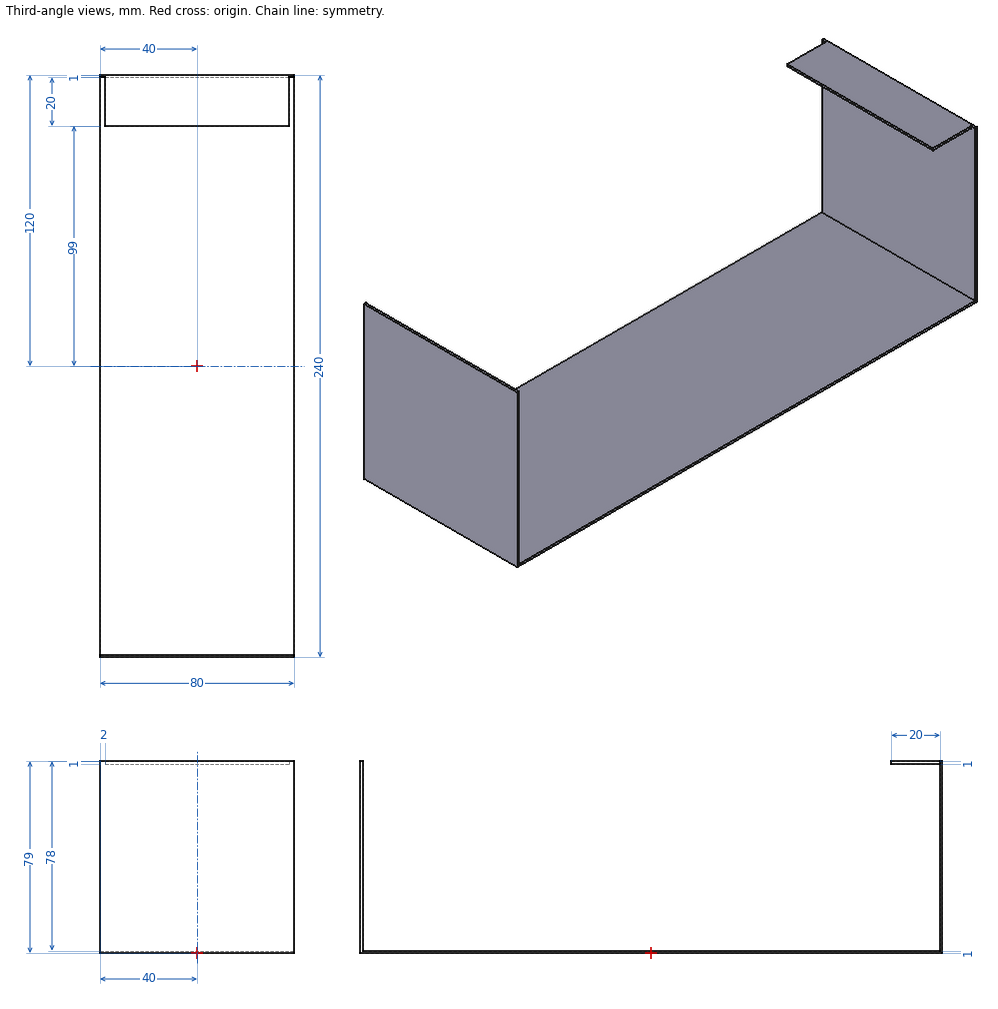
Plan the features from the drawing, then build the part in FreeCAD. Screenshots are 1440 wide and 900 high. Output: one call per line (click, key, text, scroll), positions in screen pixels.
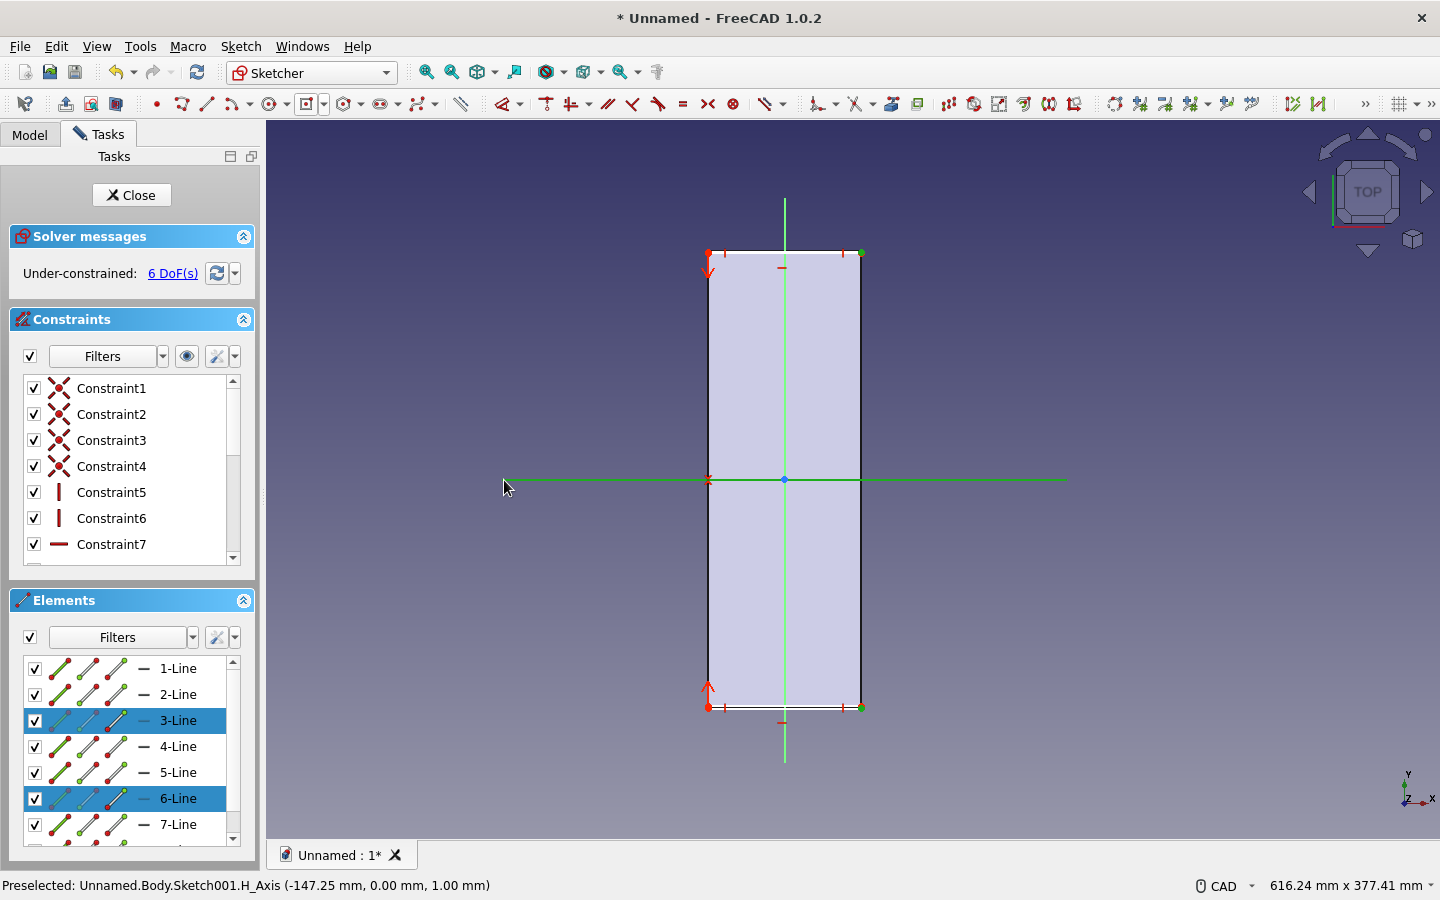
key(s)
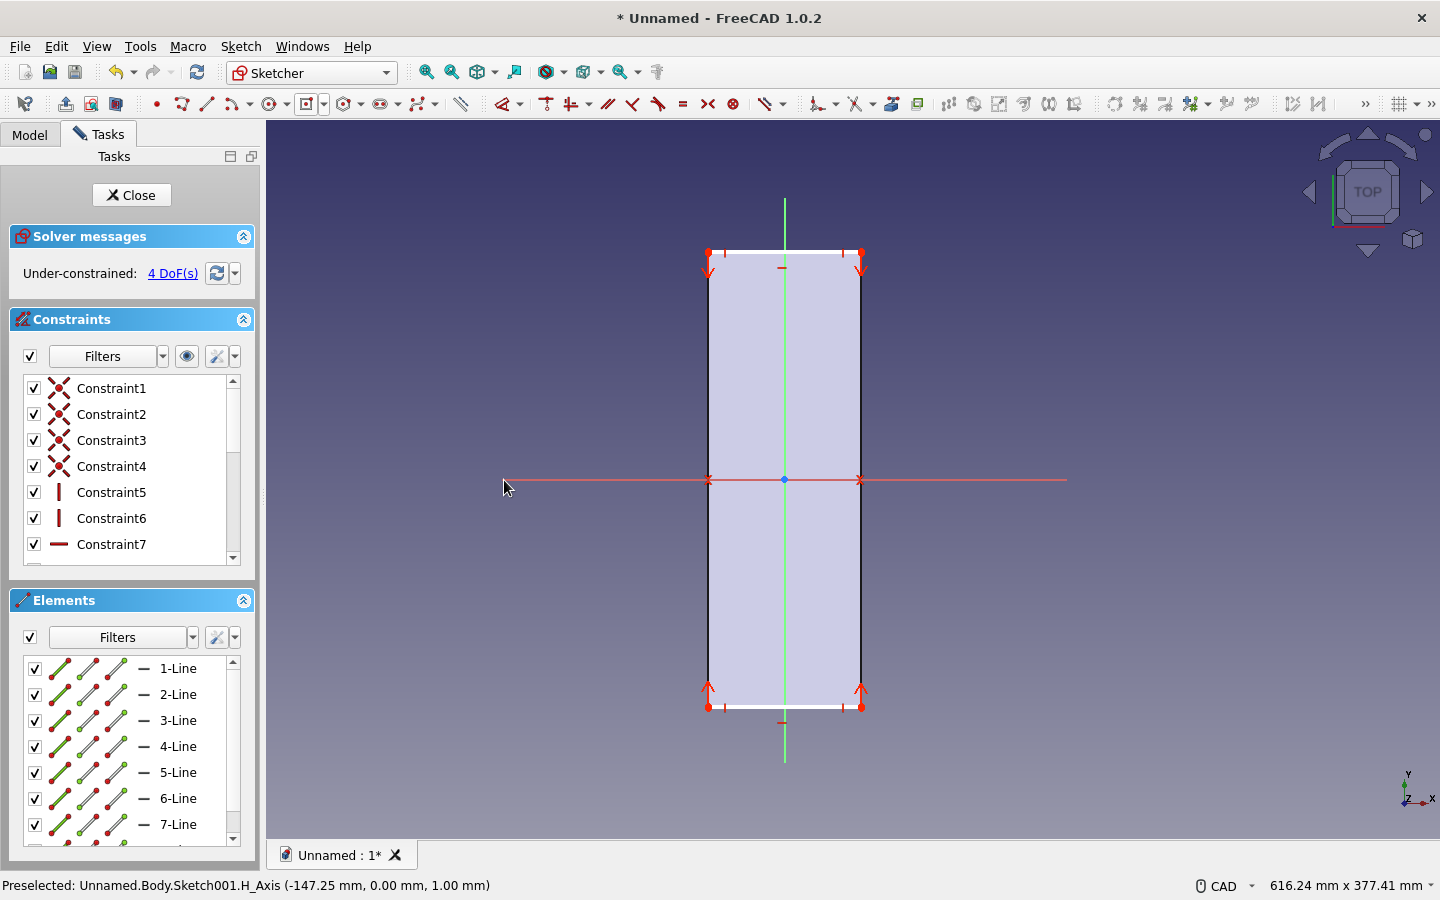
click(502, 104)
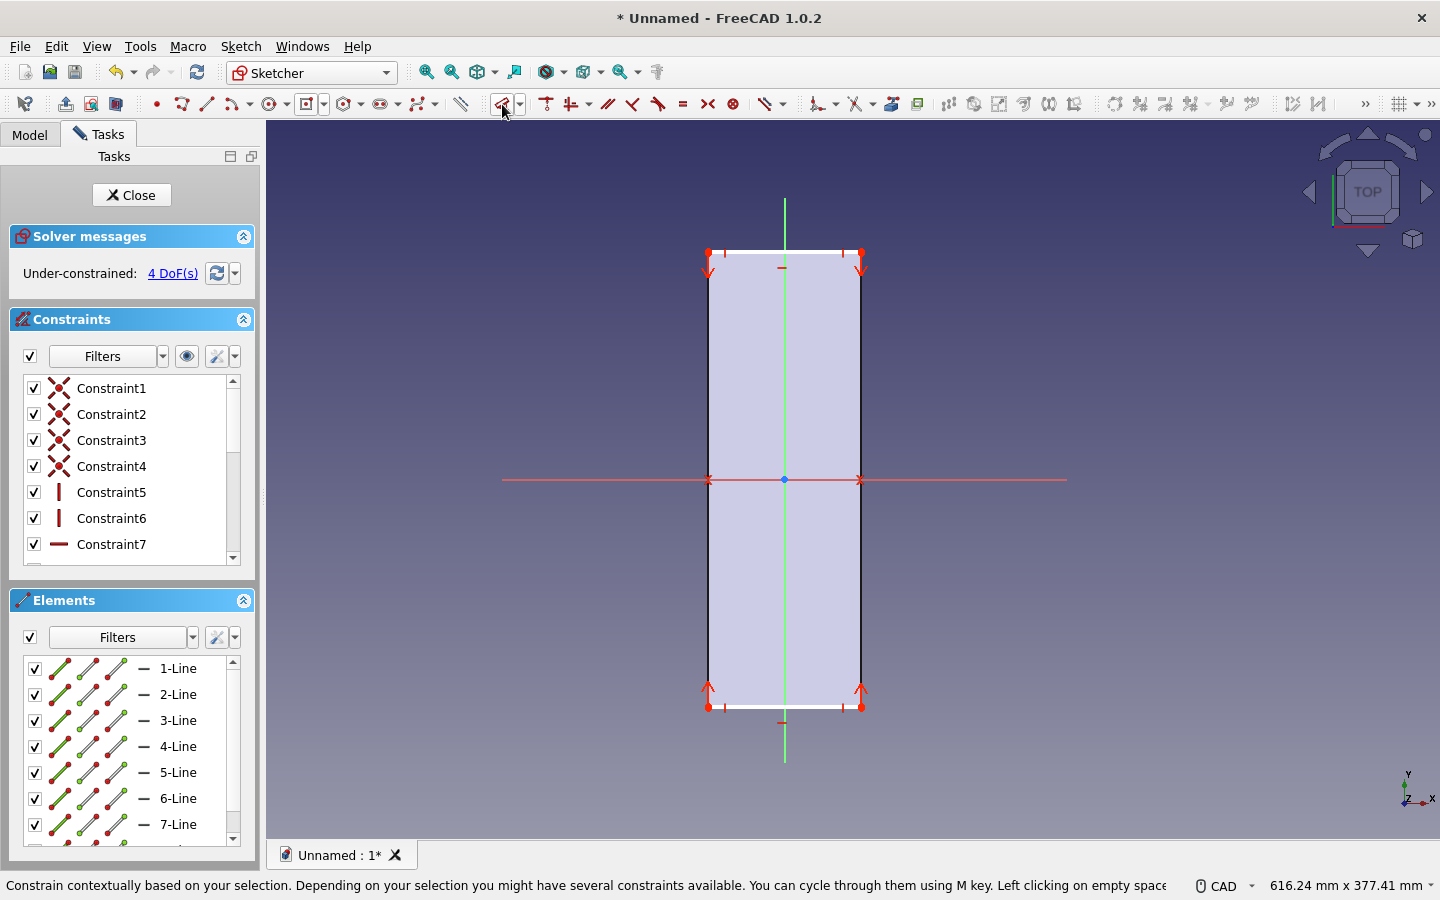
scroll(708, 252, up, 16)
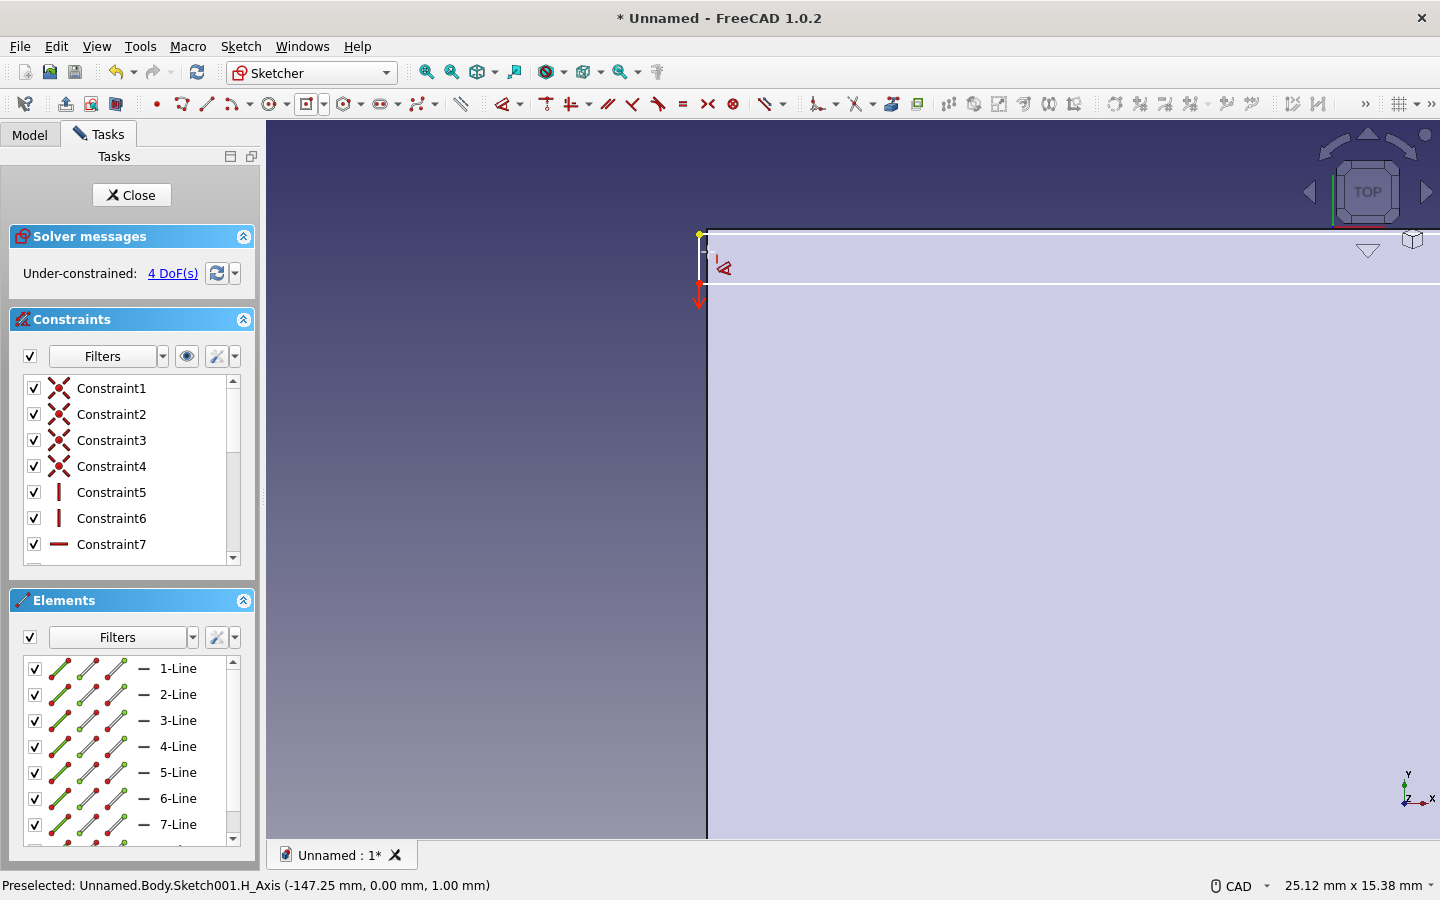
click(699, 259)
click(665, 259)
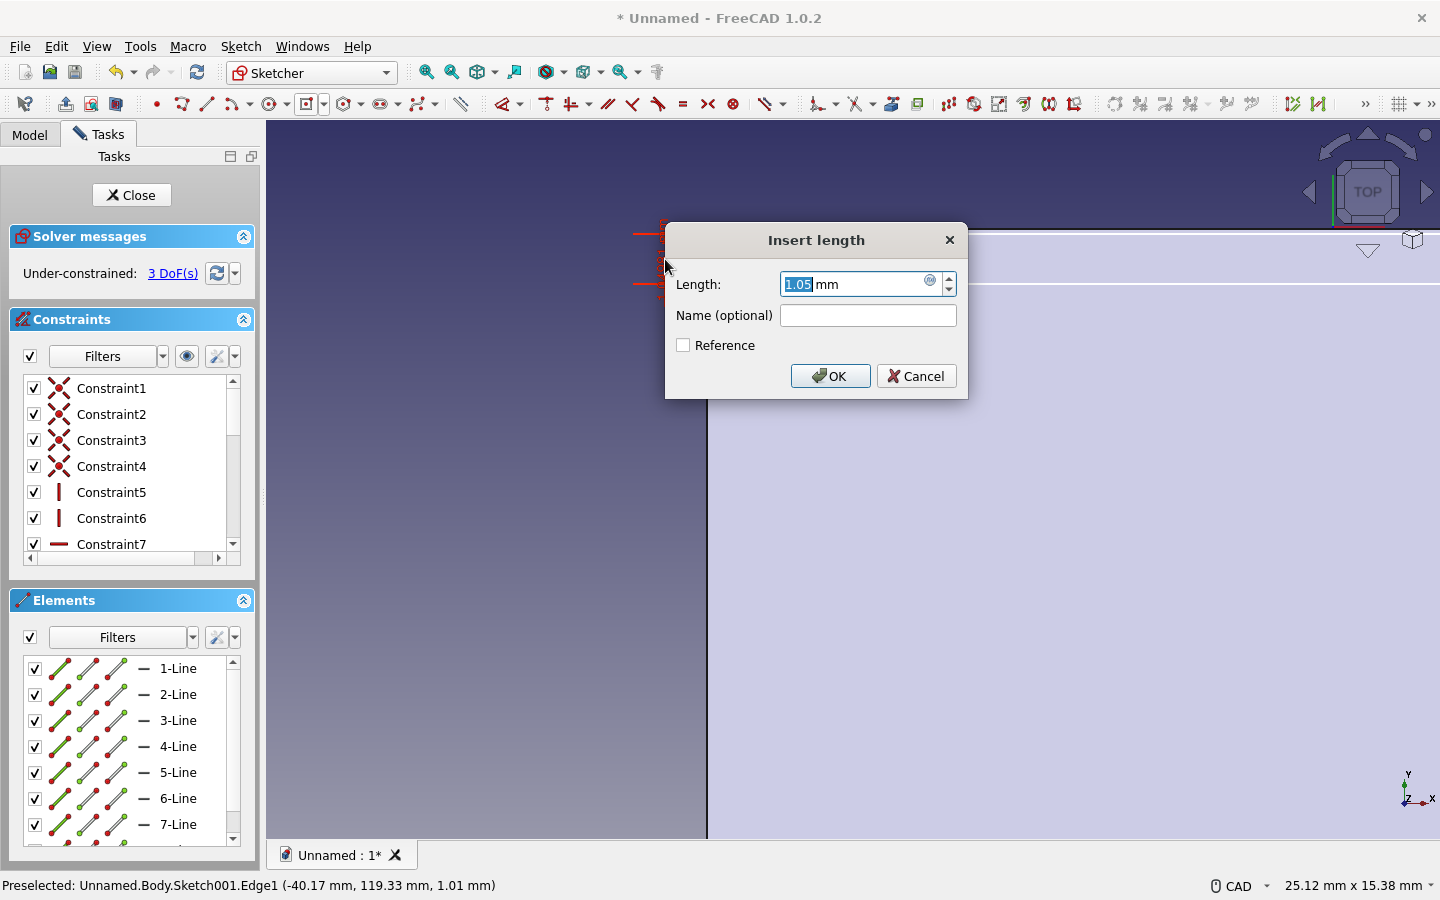
text(1)
key(Return)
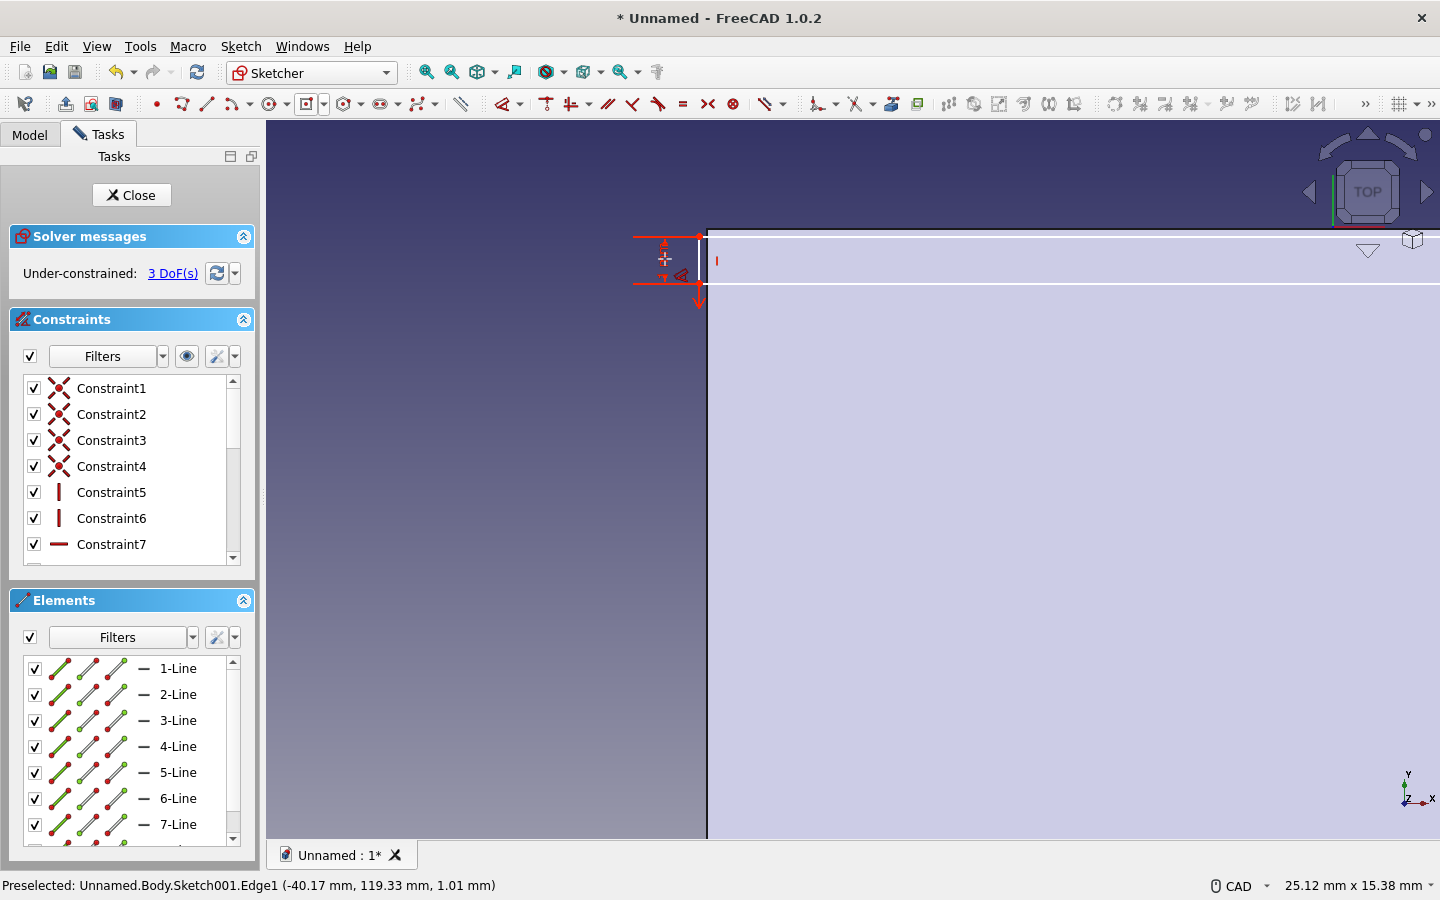
scroll(691, 199, down, 15)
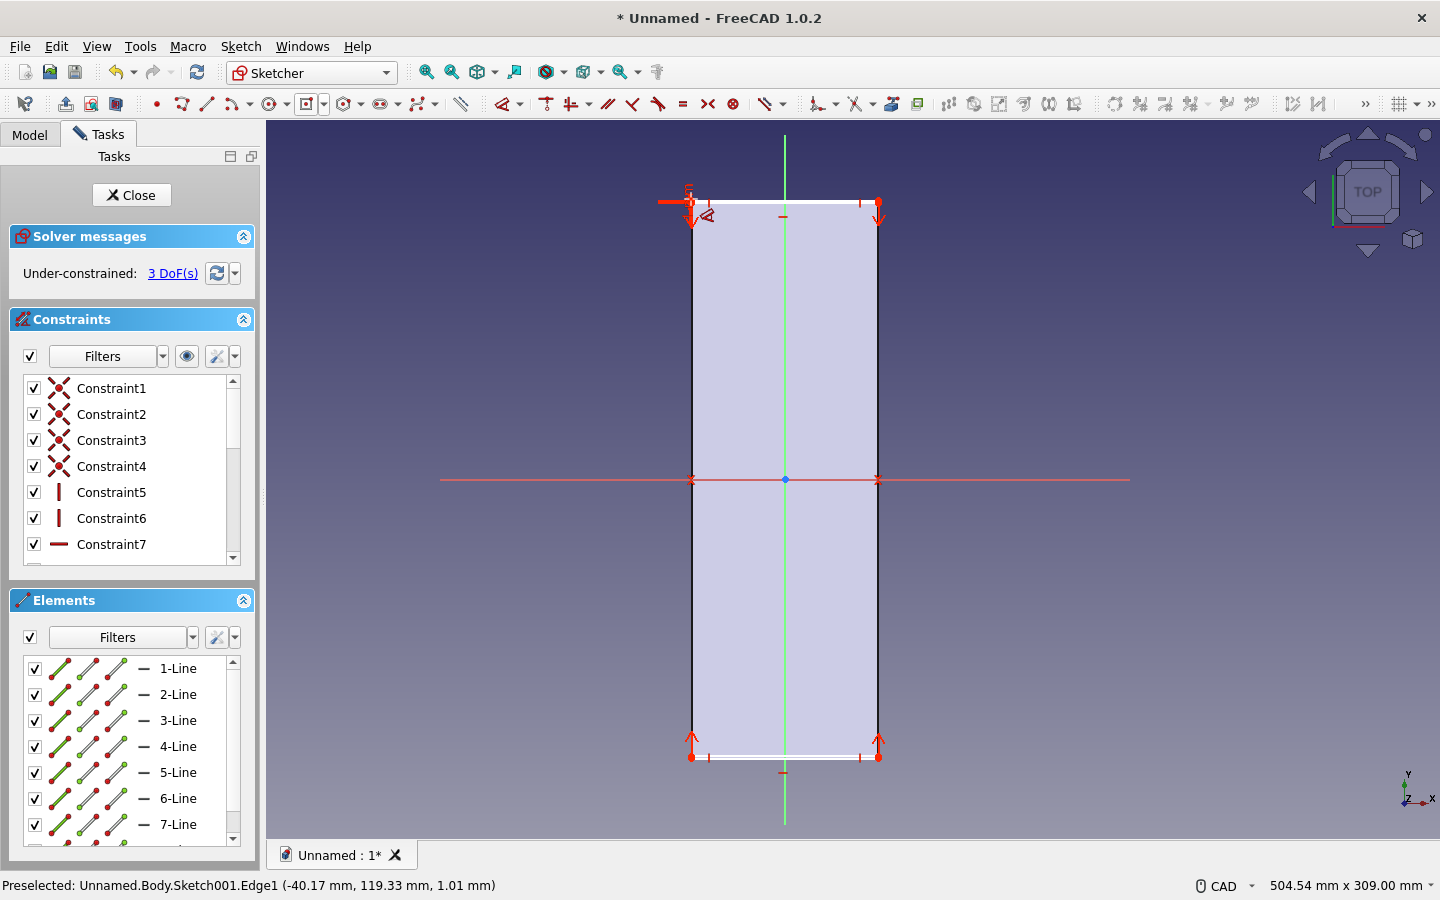
scroll(748, 203, up, 9)